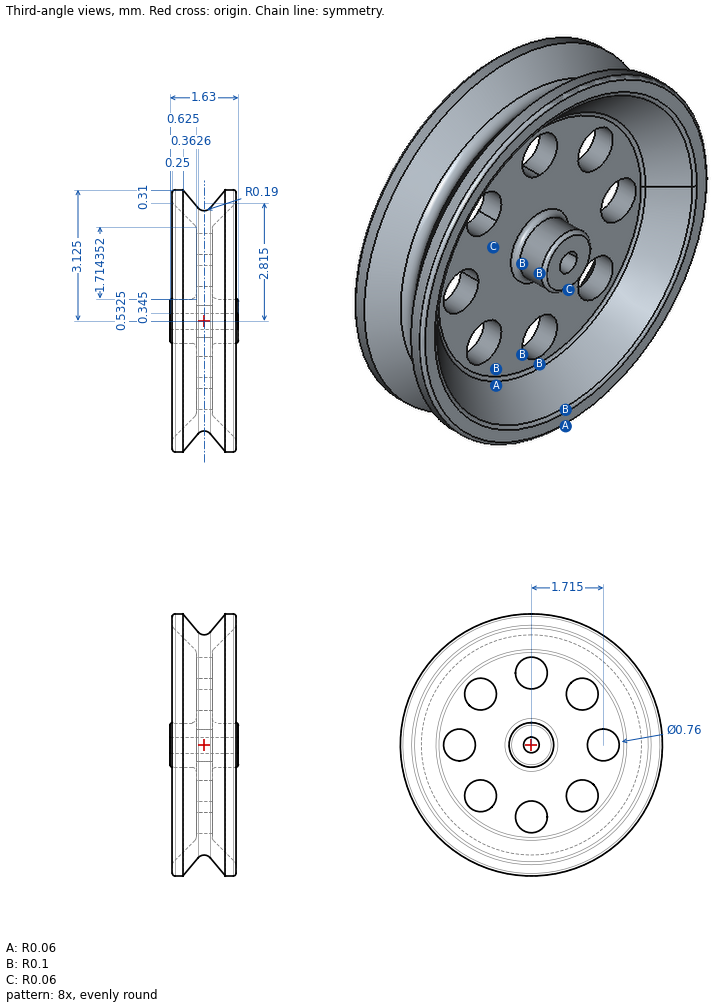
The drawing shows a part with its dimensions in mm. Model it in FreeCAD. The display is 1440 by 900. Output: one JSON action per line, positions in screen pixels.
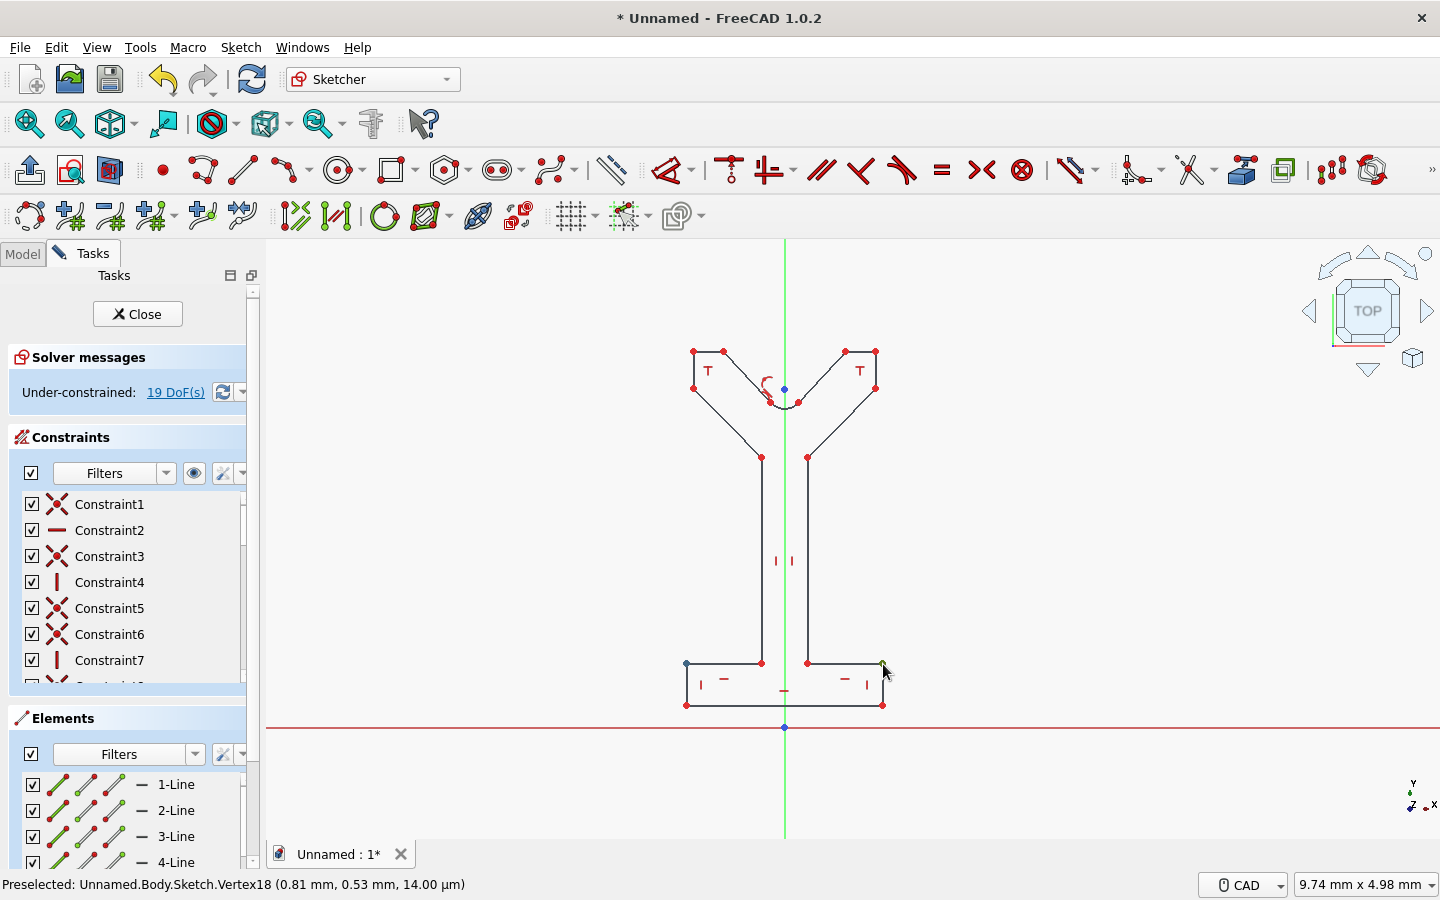
{"action": "left_click", "coordinate": [785, 772]}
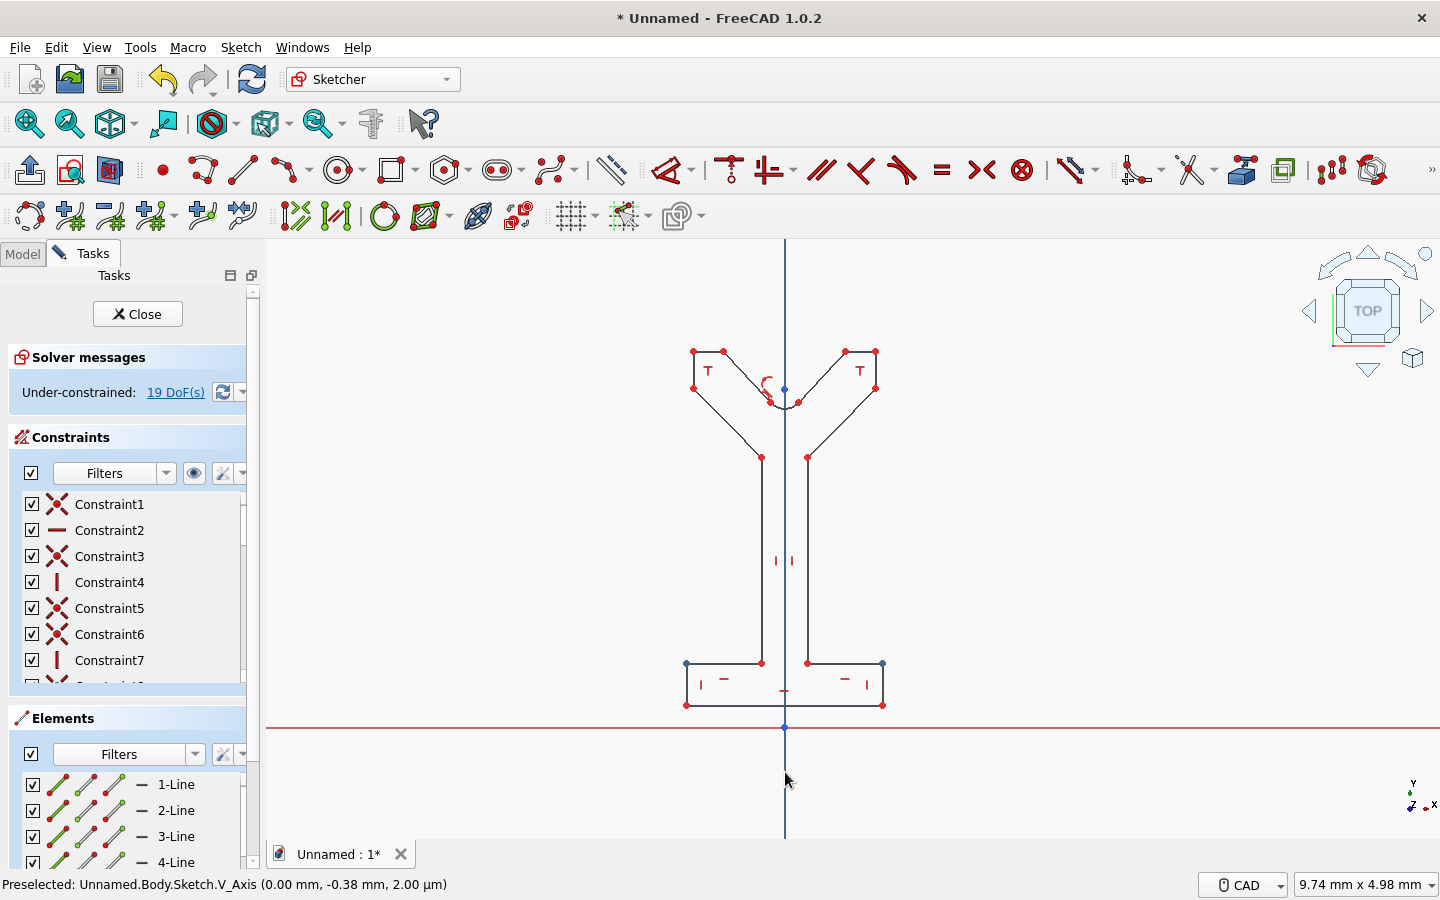
{"action": "left_click", "coordinate": [982, 170]}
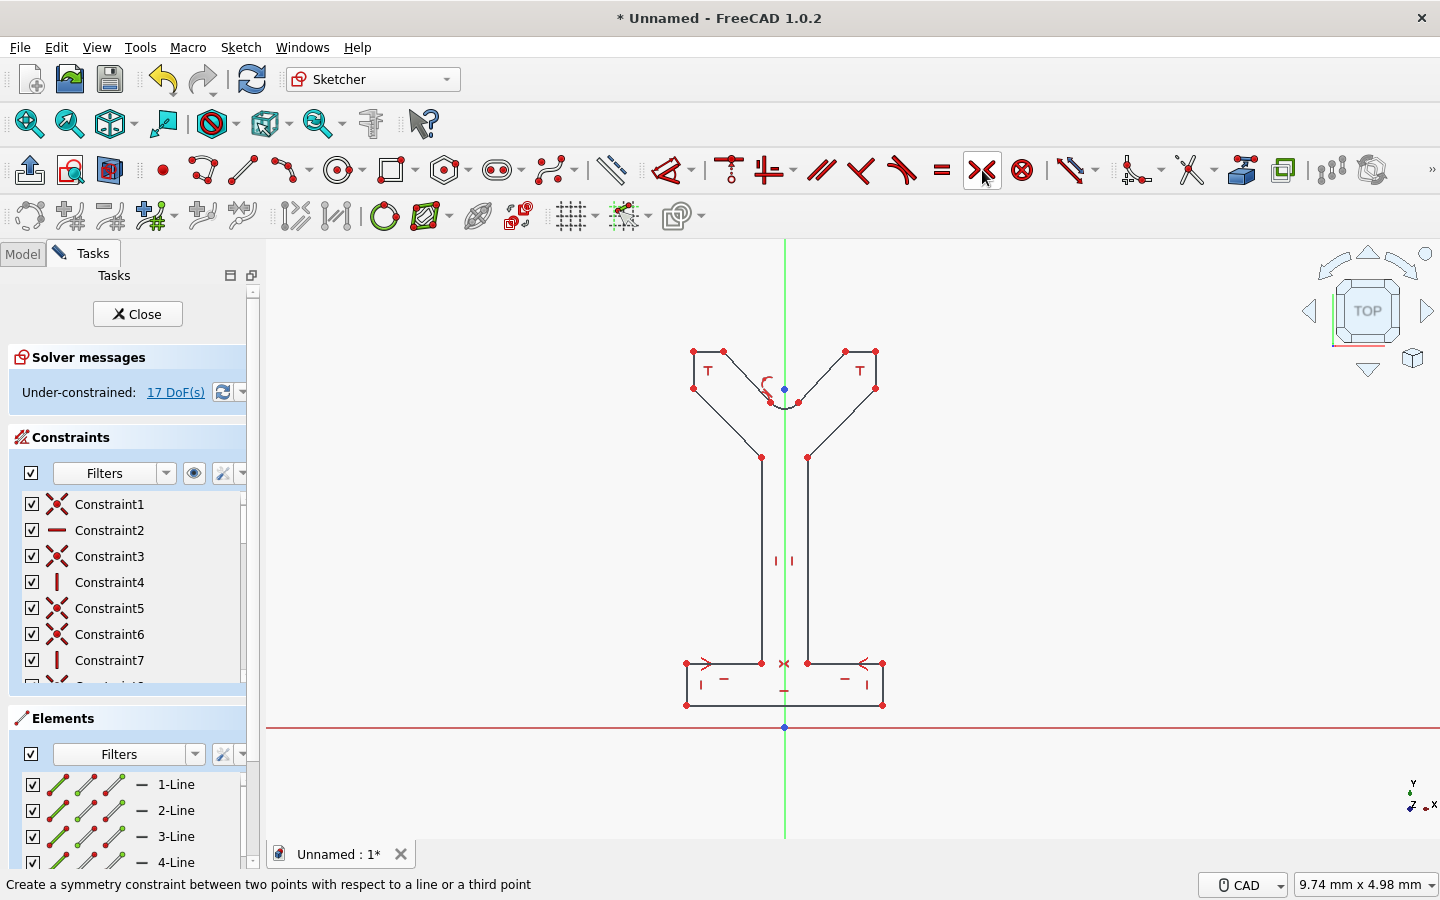
{"action": "left_click", "coordinate": [762, 458]}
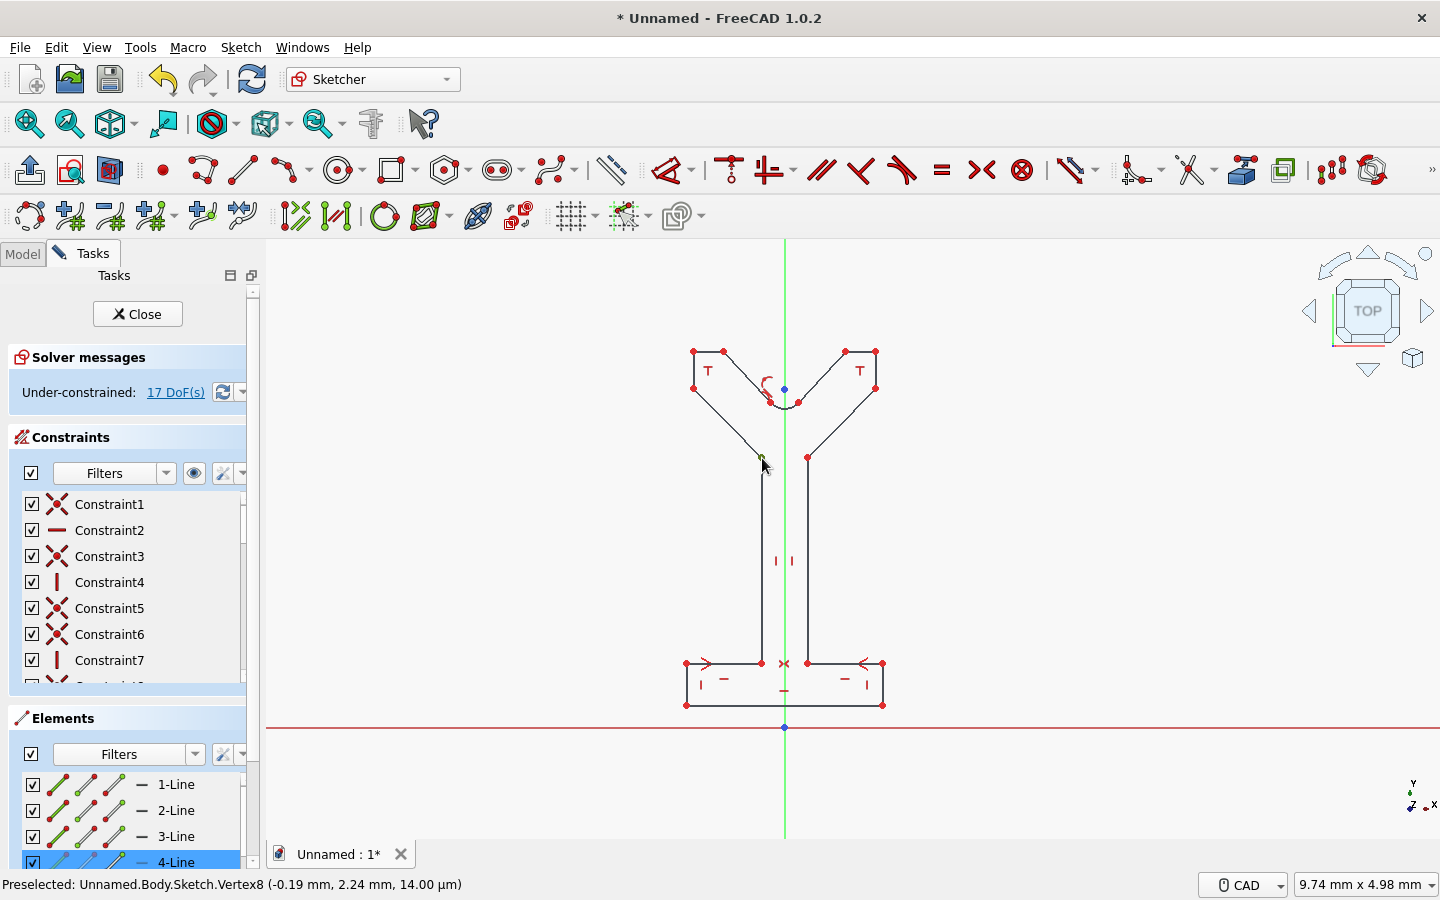
{"action": "left_click", "coordinate": [808, 458]}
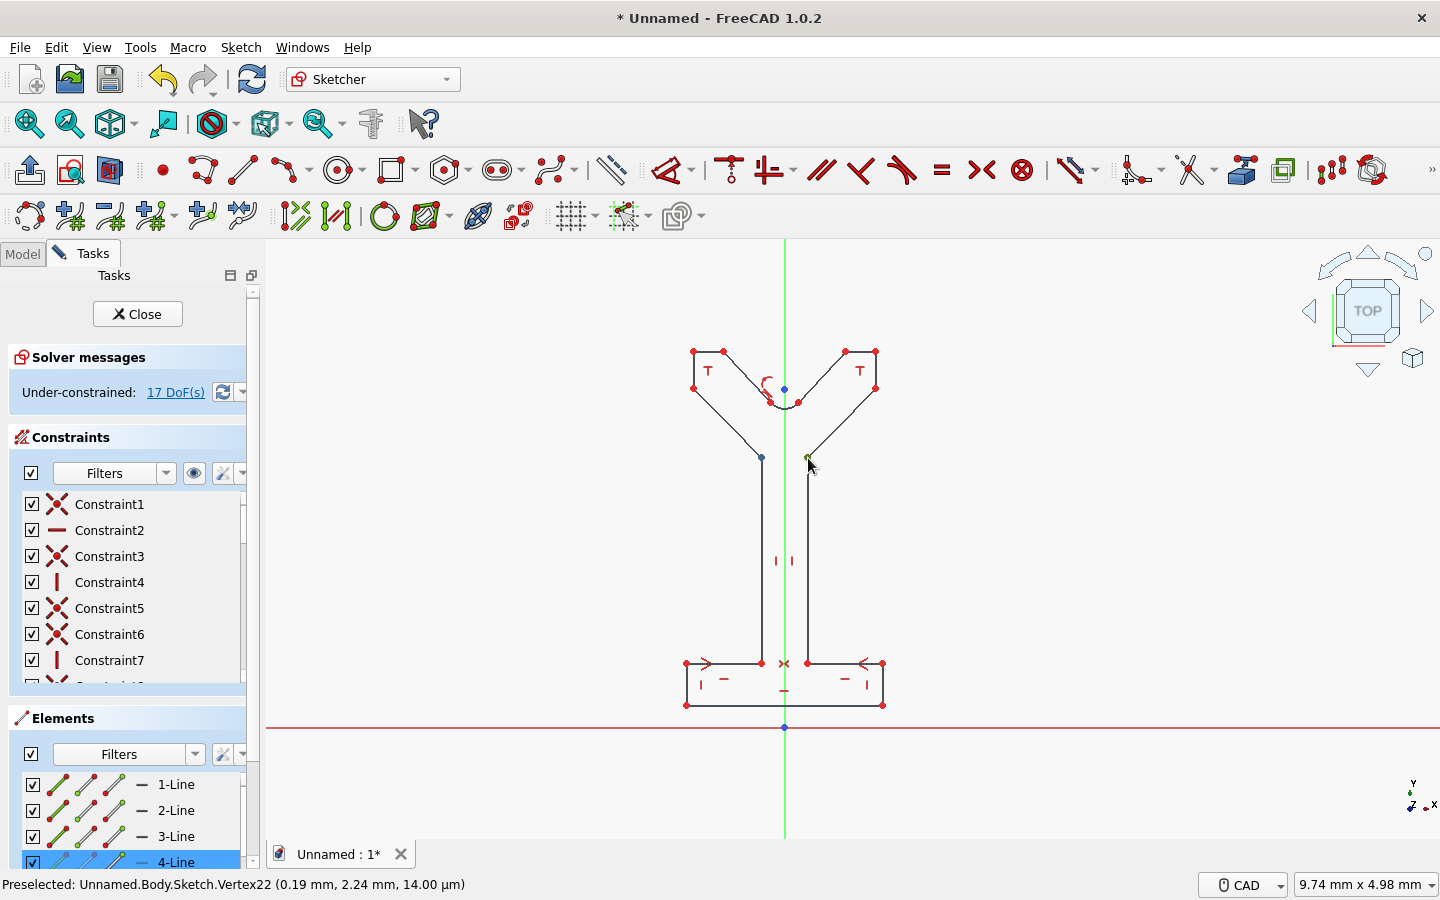
{"action": "left_click", "coordinate": [785, 772]}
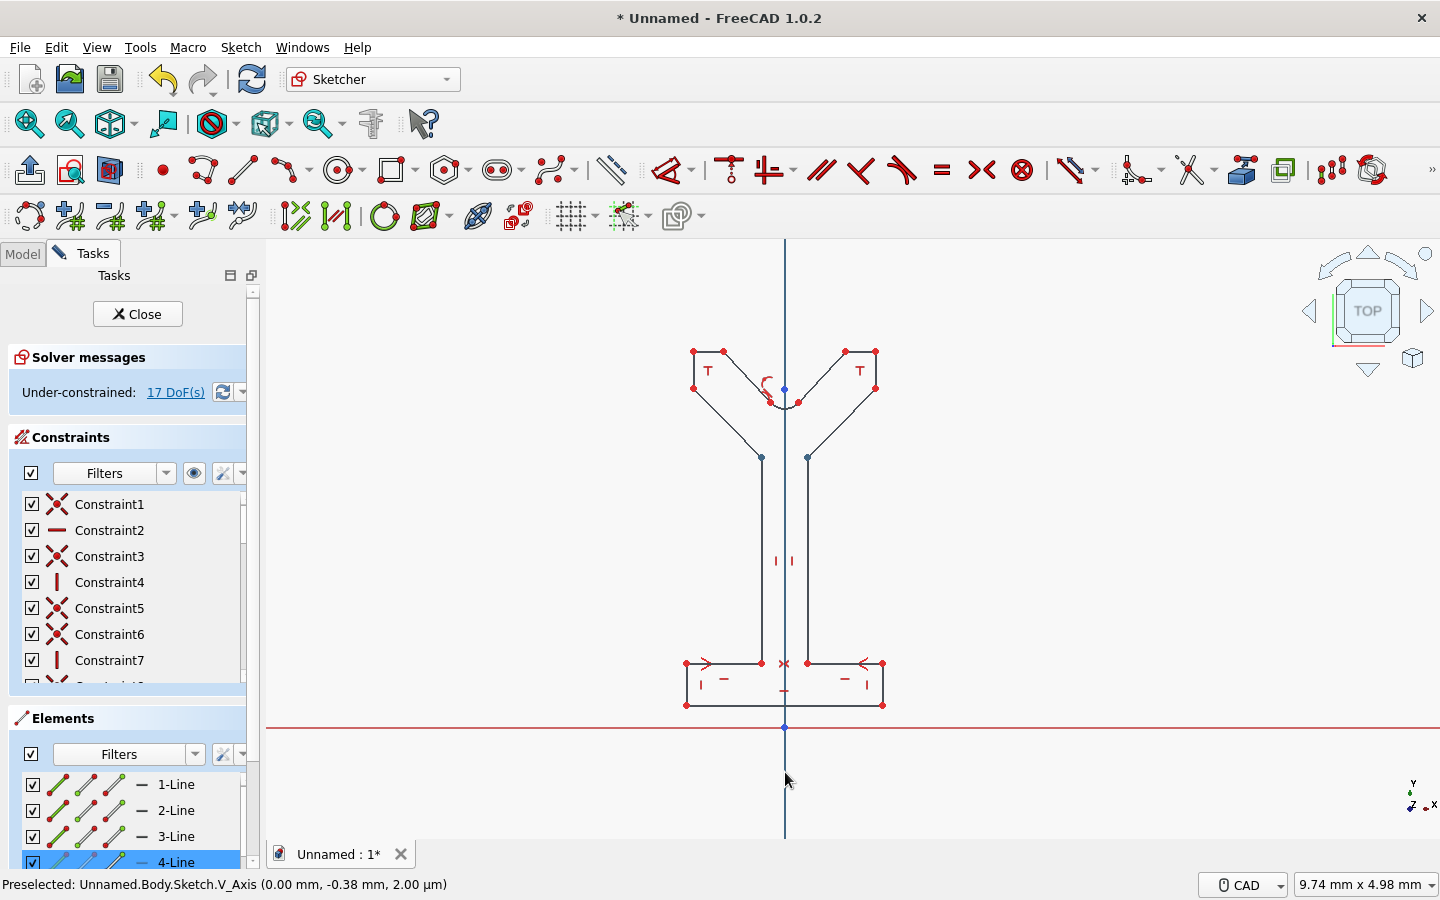
{"action": "left_click", "coordinate": [982, 170]}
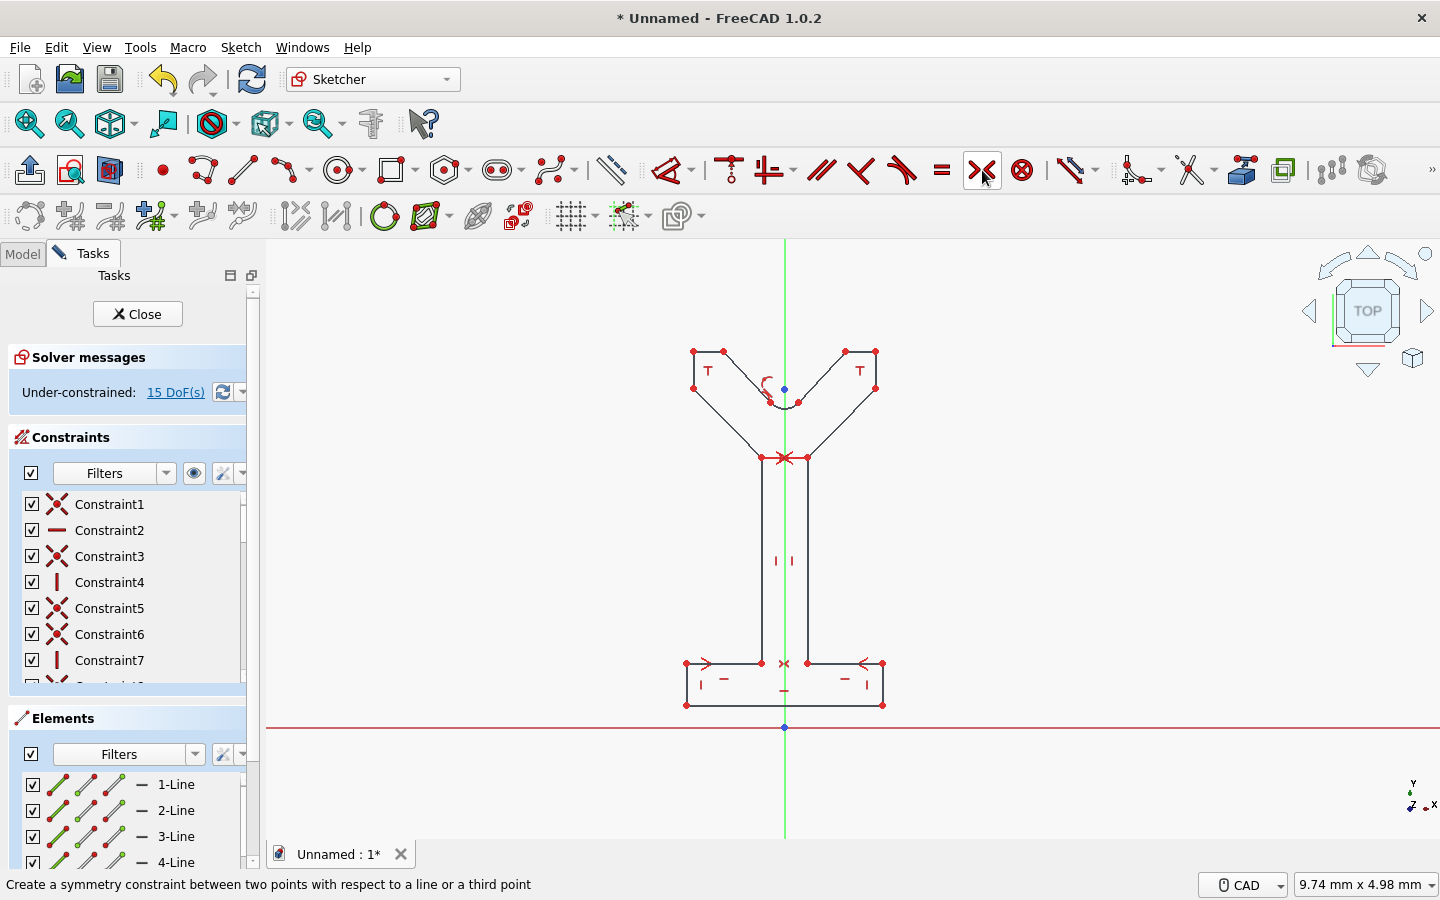
{"action": "left_click", "coordinate": [694, 389]}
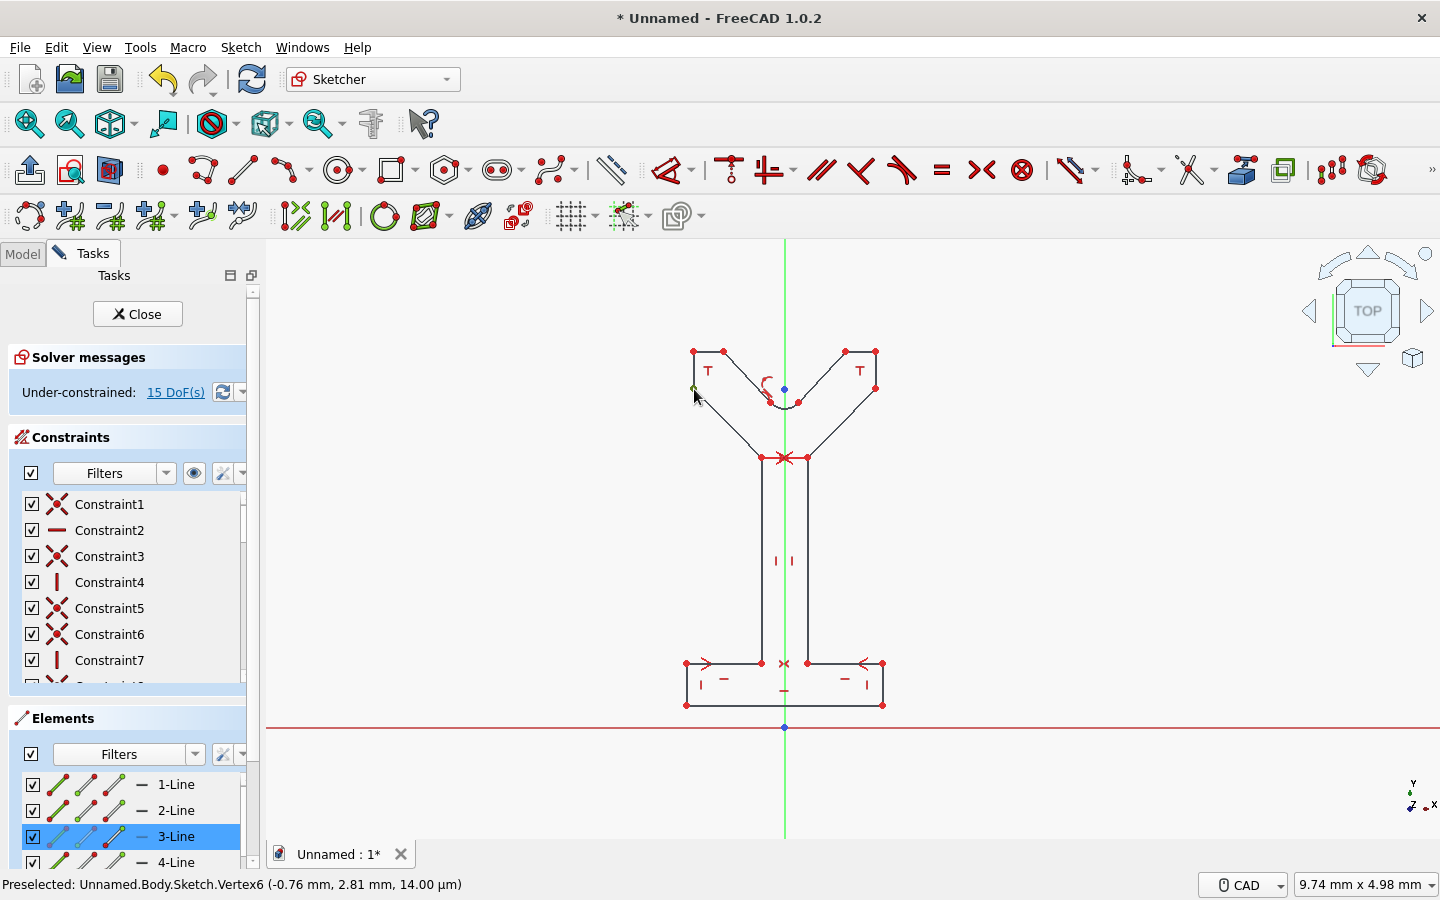
{"action": "left_click", "coordinate": [876, 389]}